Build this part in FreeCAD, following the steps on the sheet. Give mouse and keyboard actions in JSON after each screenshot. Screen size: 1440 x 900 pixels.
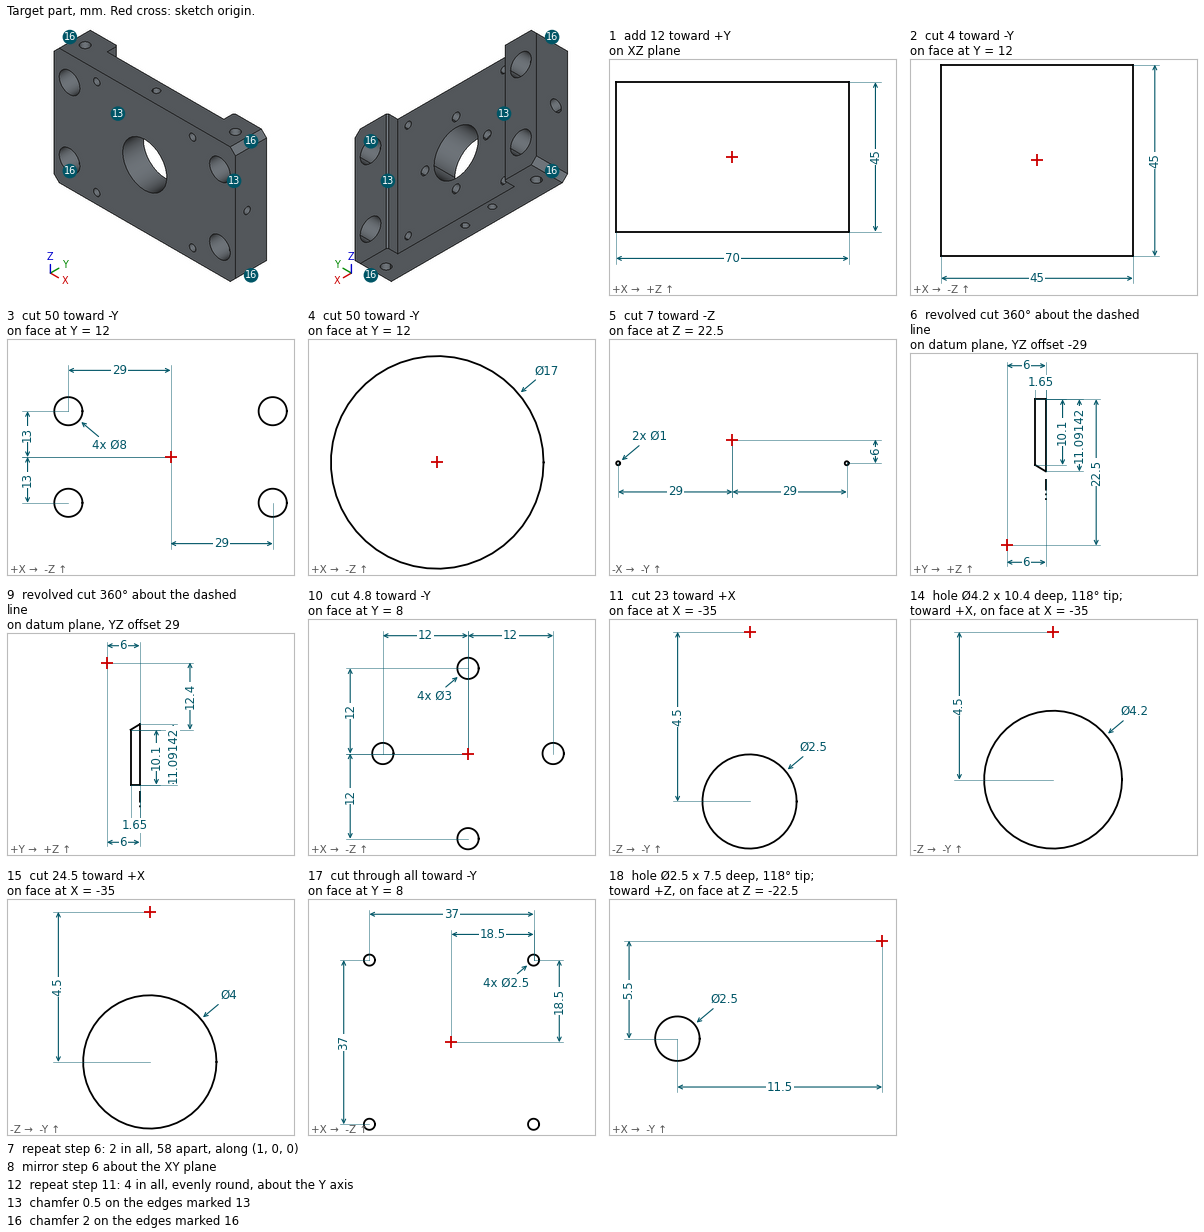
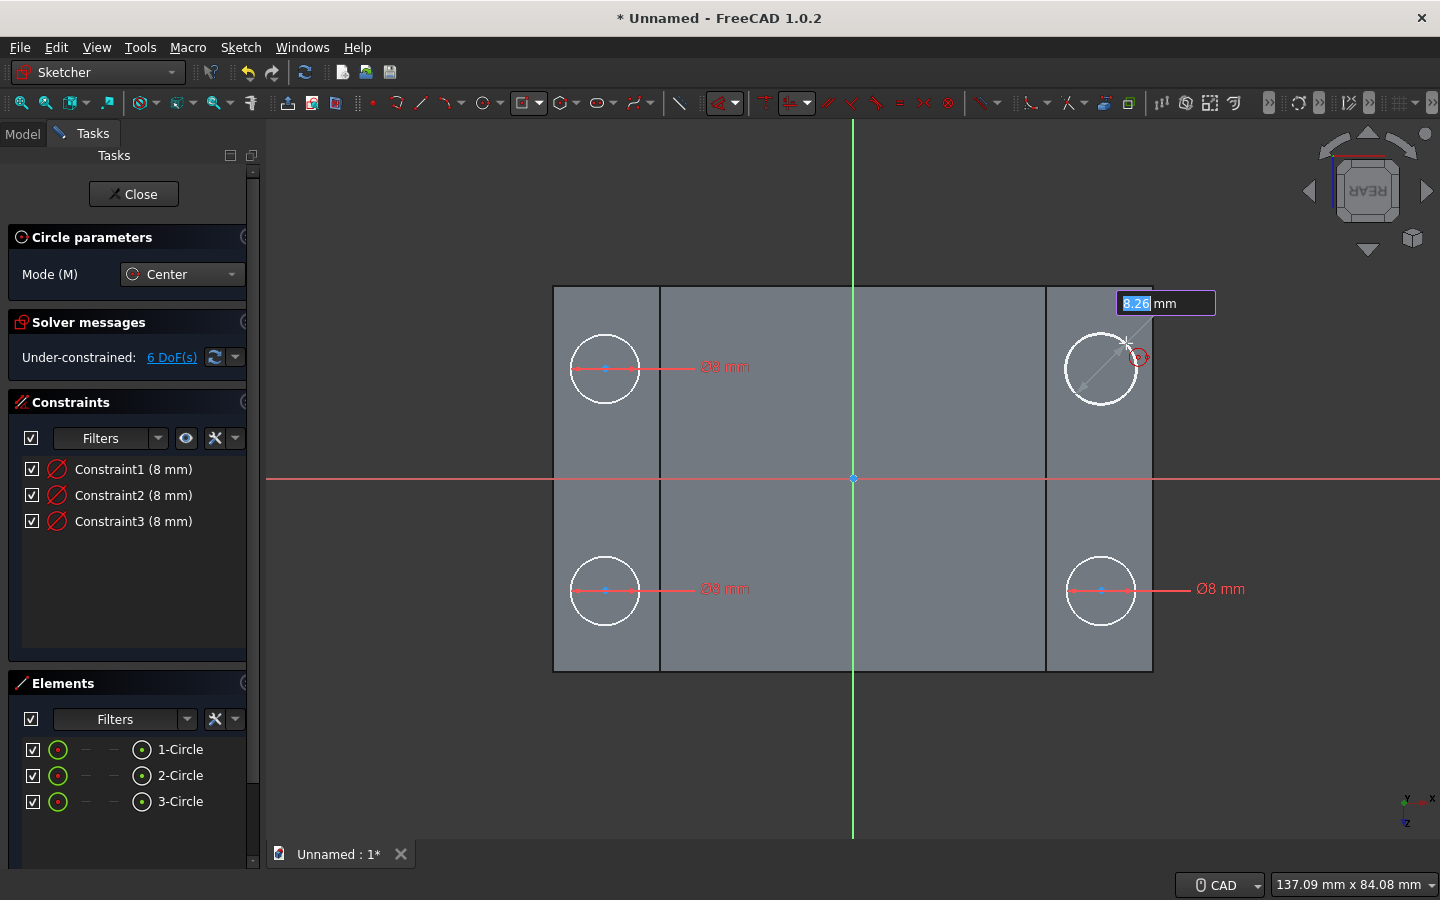
{"action": "type", "text": "8"}
{"action": "key", "text": "Return"}
{"action": "key", "text": "Escape"}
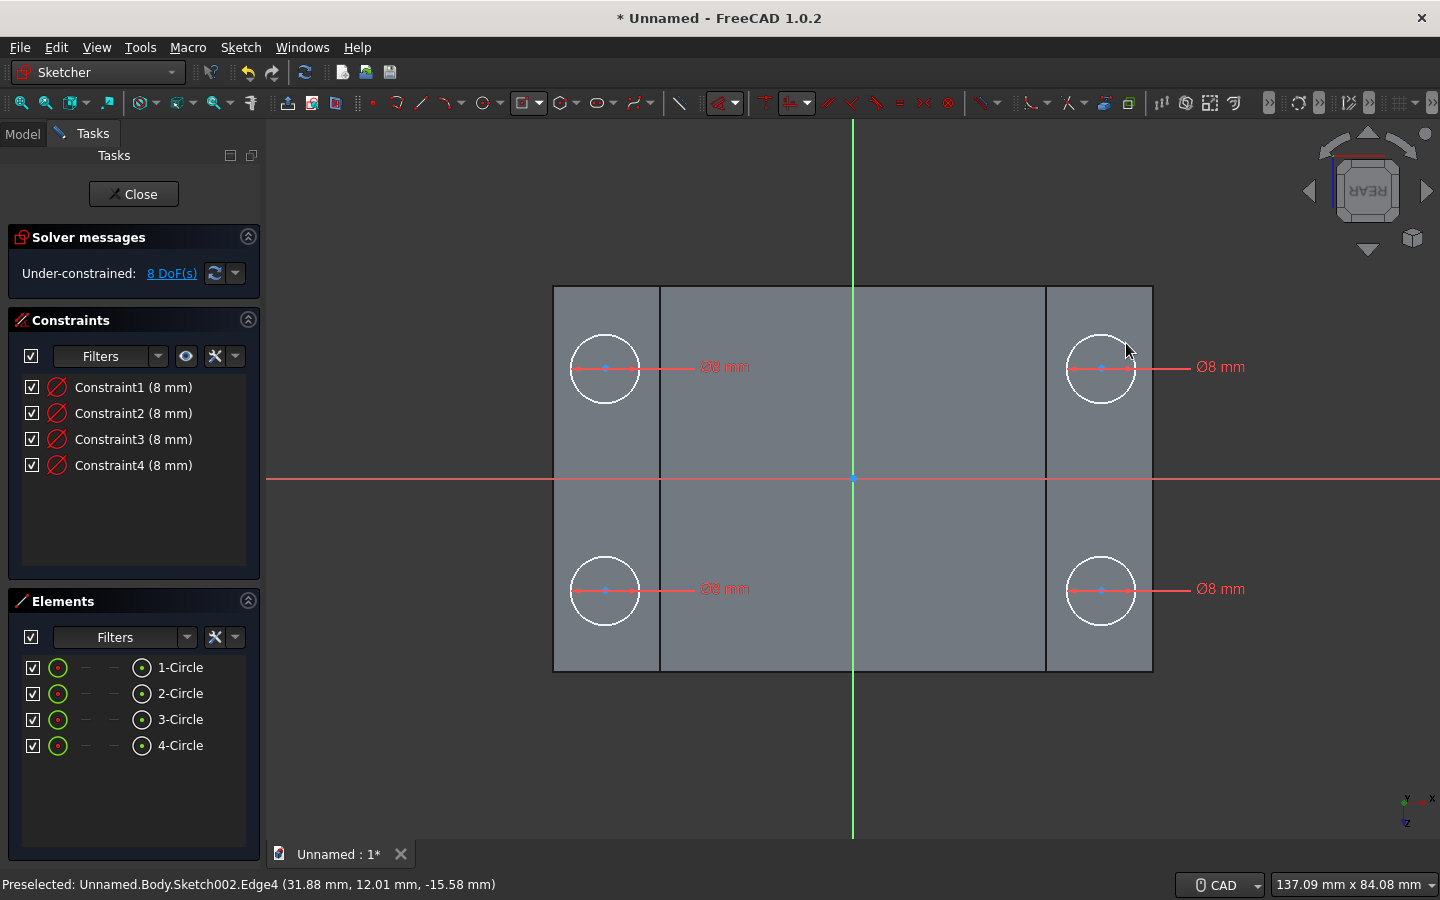
{"action": "left_click", "coordinate": [605, 369]}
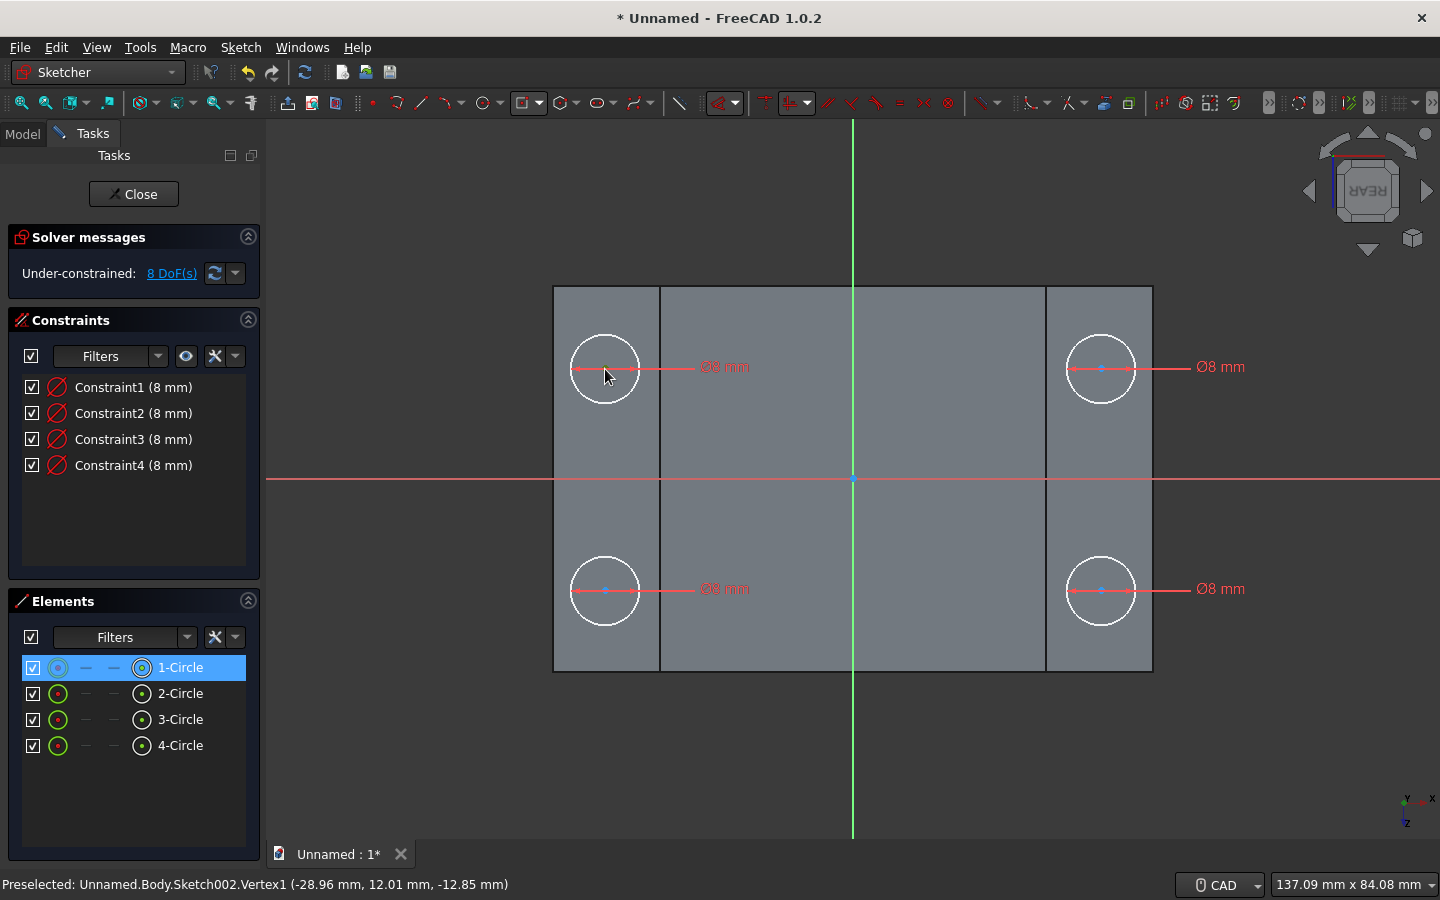
{"action": "left_click", "coordinate": [605, 591]}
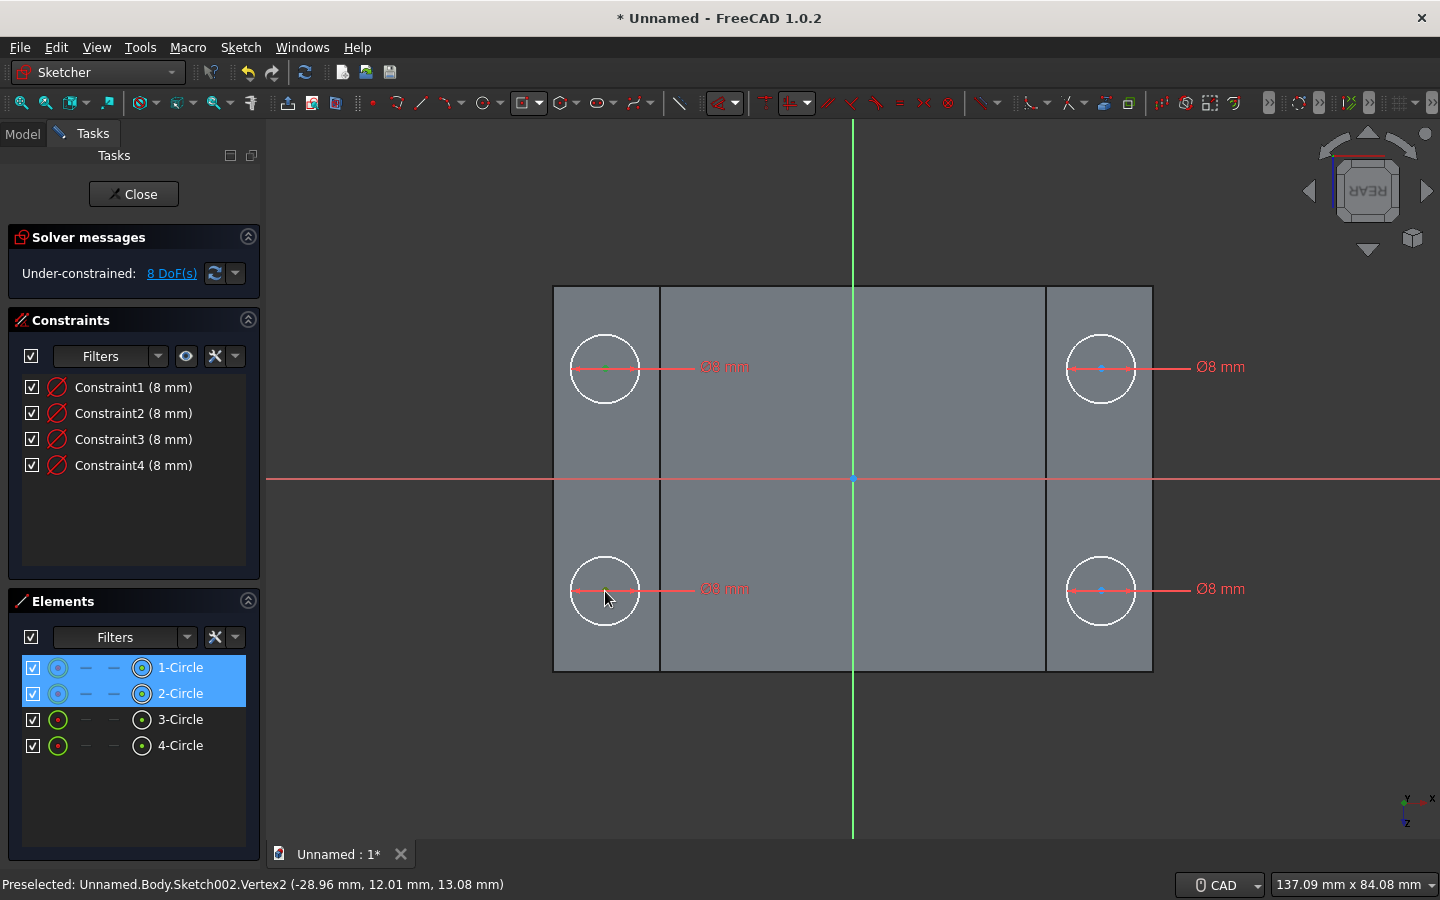
{"action": "left_click", "coordinate": [810, 104]}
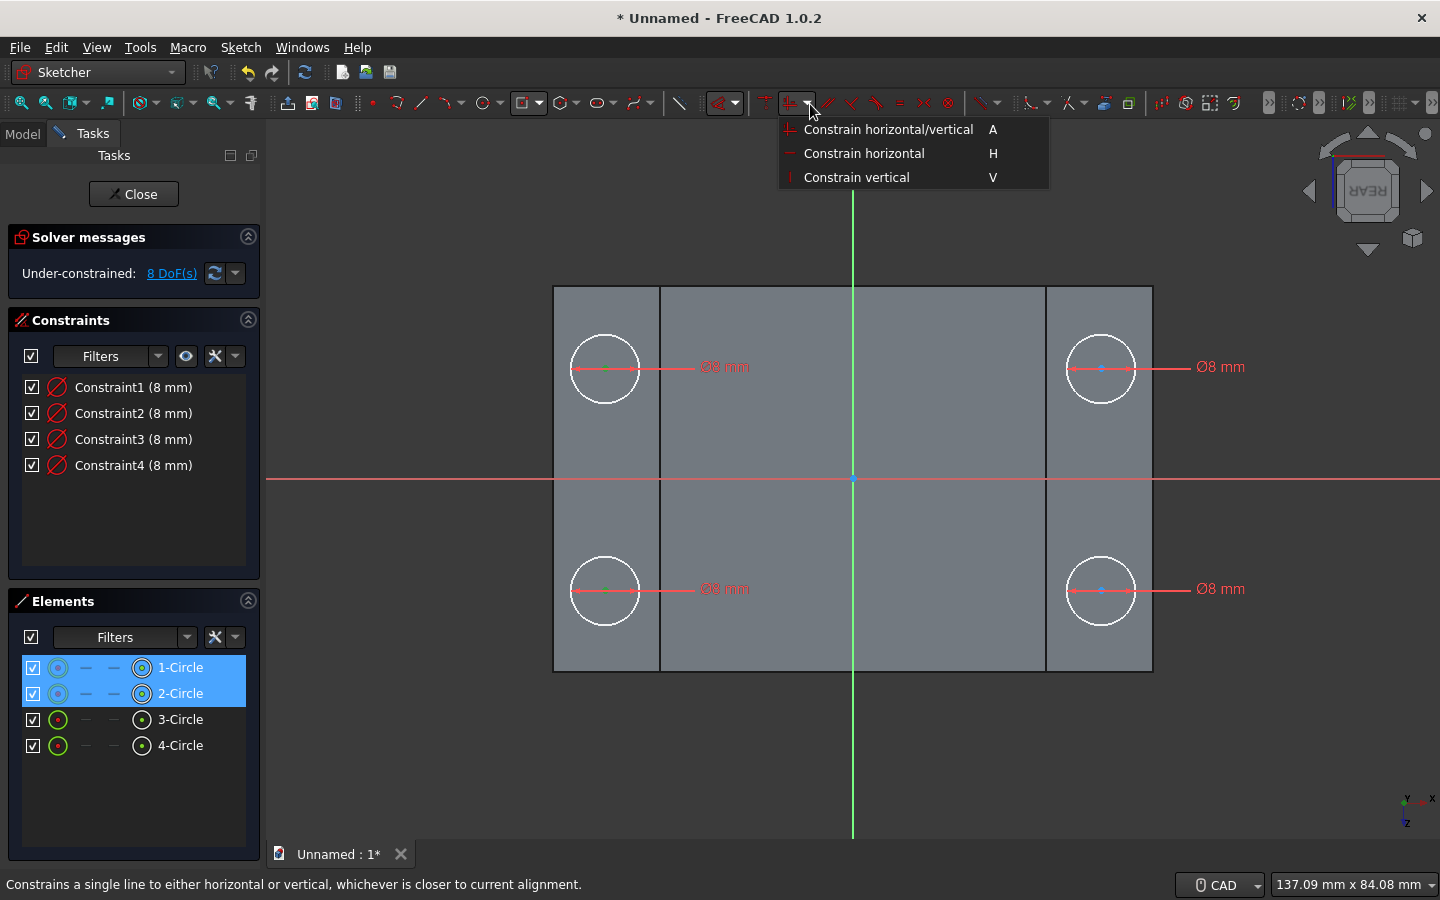
{"action": "left_click", "coordinate": [914, 177]}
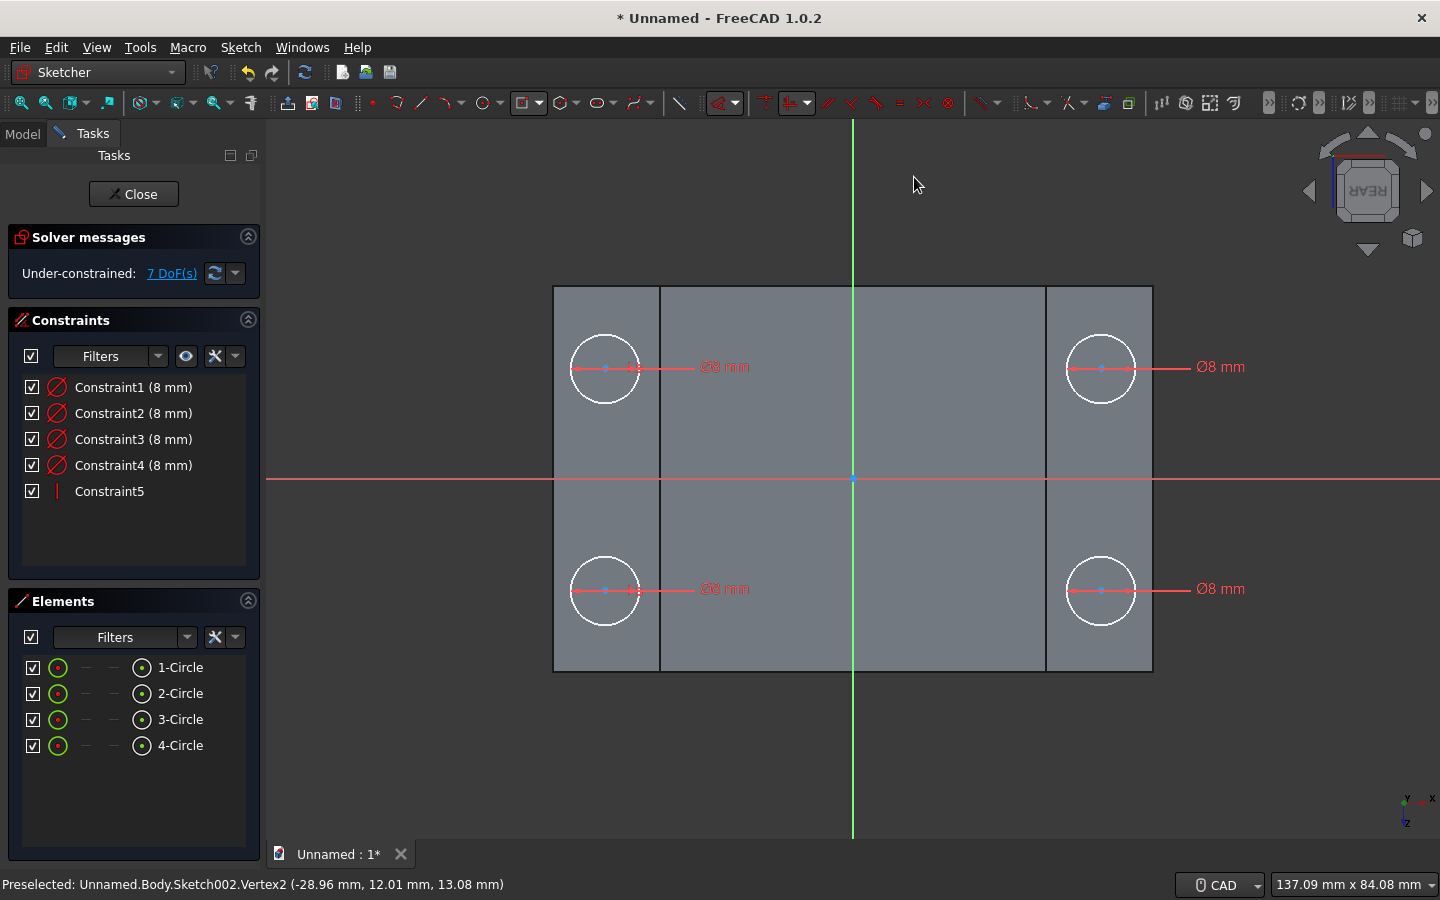
{"action": "left_click", "coordinate": [605, 591]}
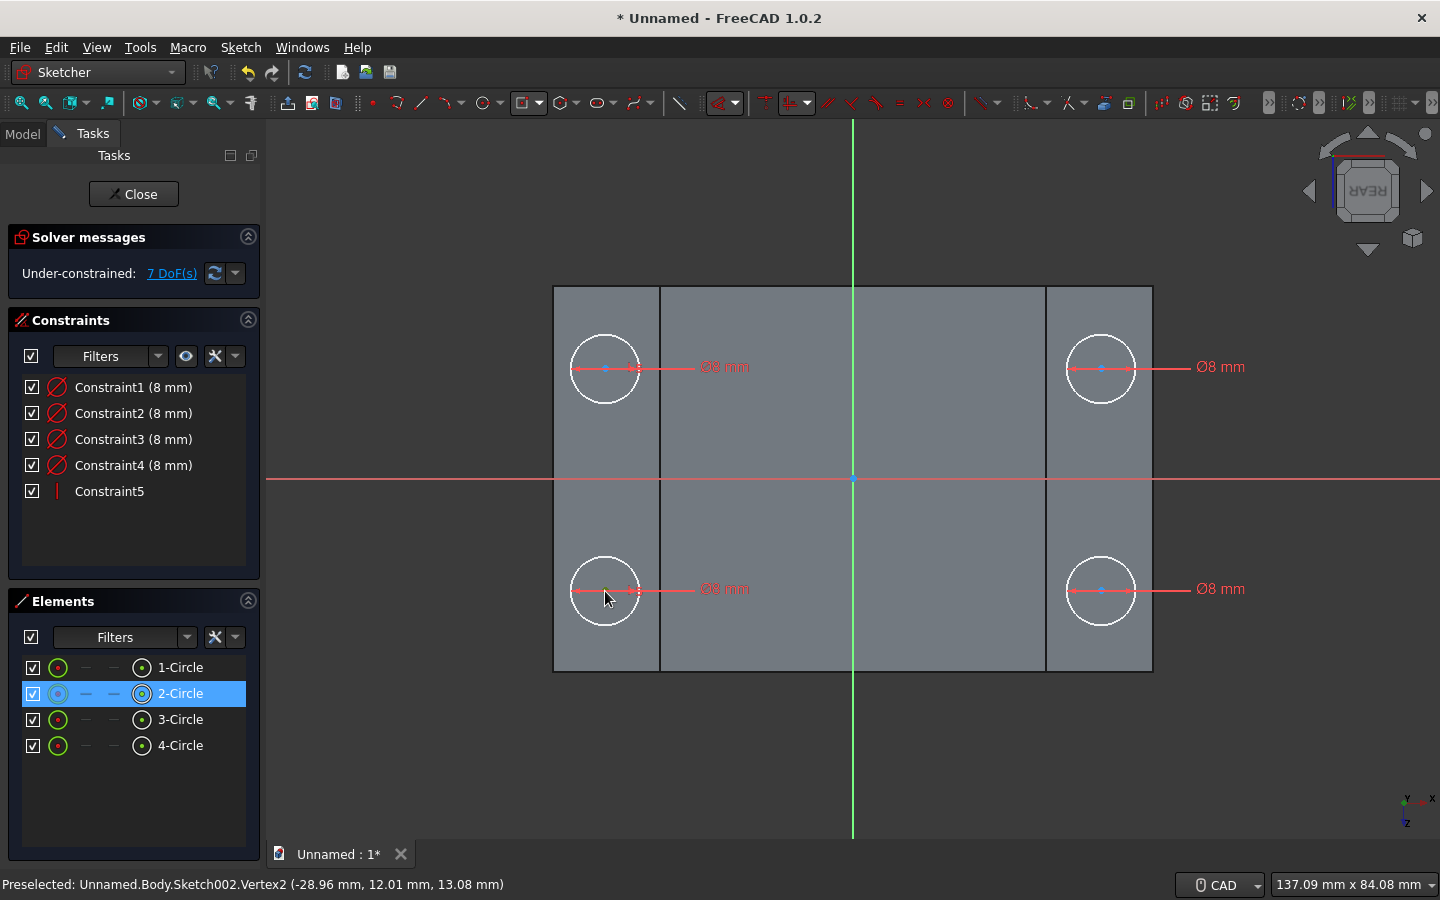
{"action": "left_click", "coordinate": [1101, 591]}